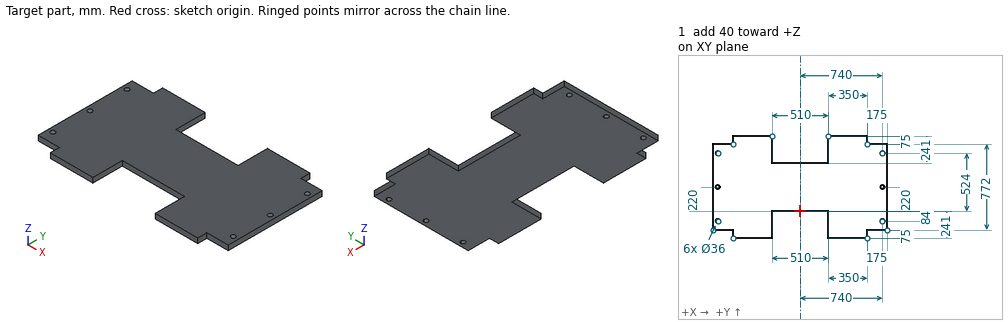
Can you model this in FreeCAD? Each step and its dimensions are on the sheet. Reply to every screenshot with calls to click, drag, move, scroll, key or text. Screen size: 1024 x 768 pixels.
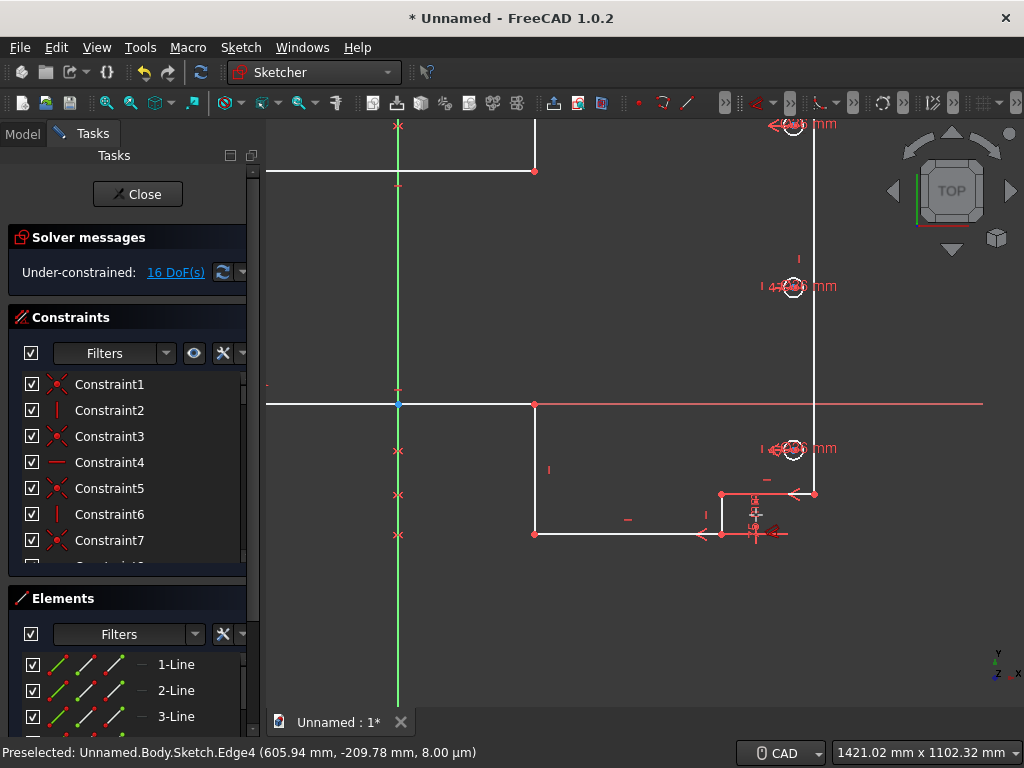
scroll(722, 516, down, 4)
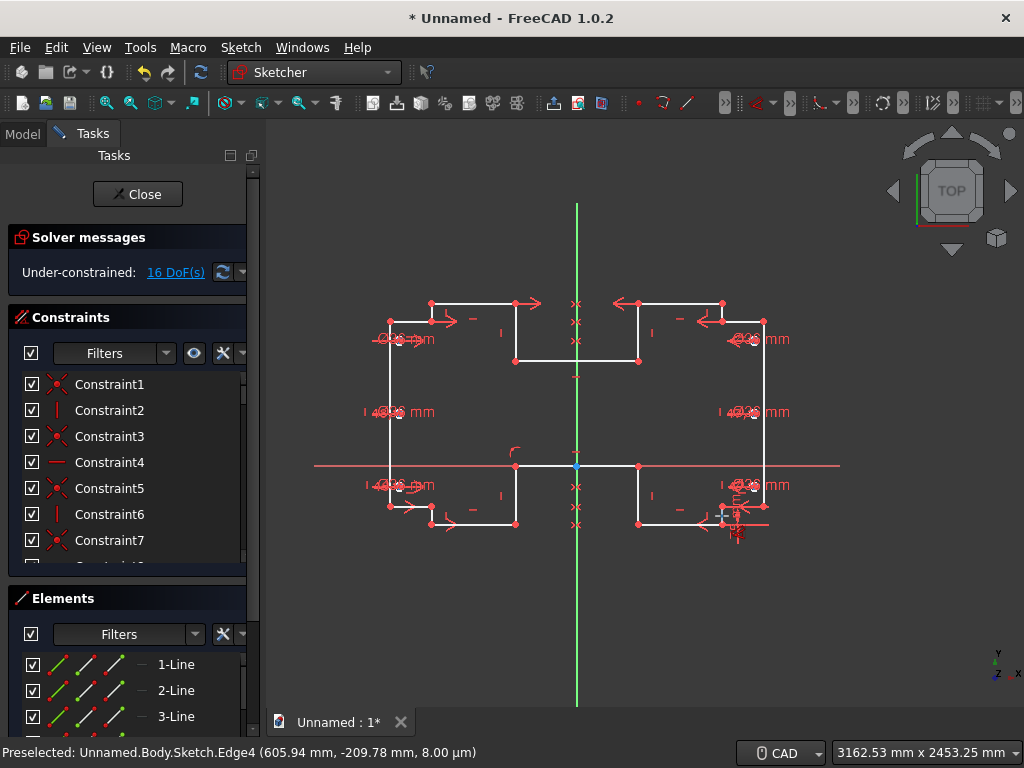
scroll(722, 316, up, 5)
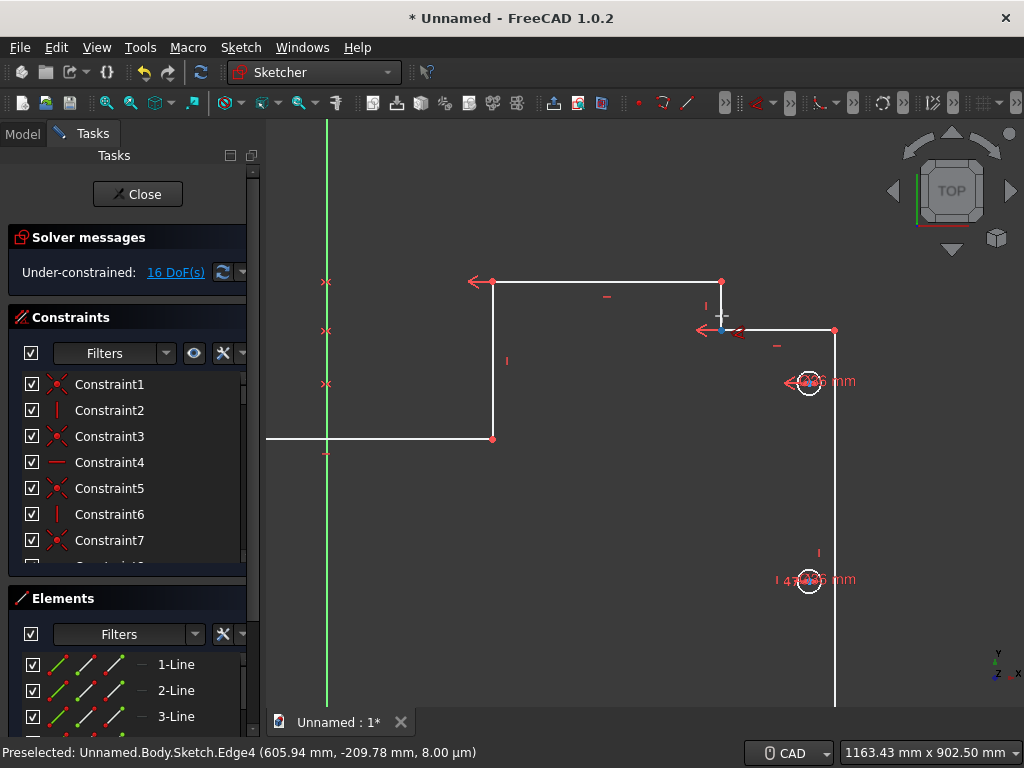
click(721, 316)
click(755, 306)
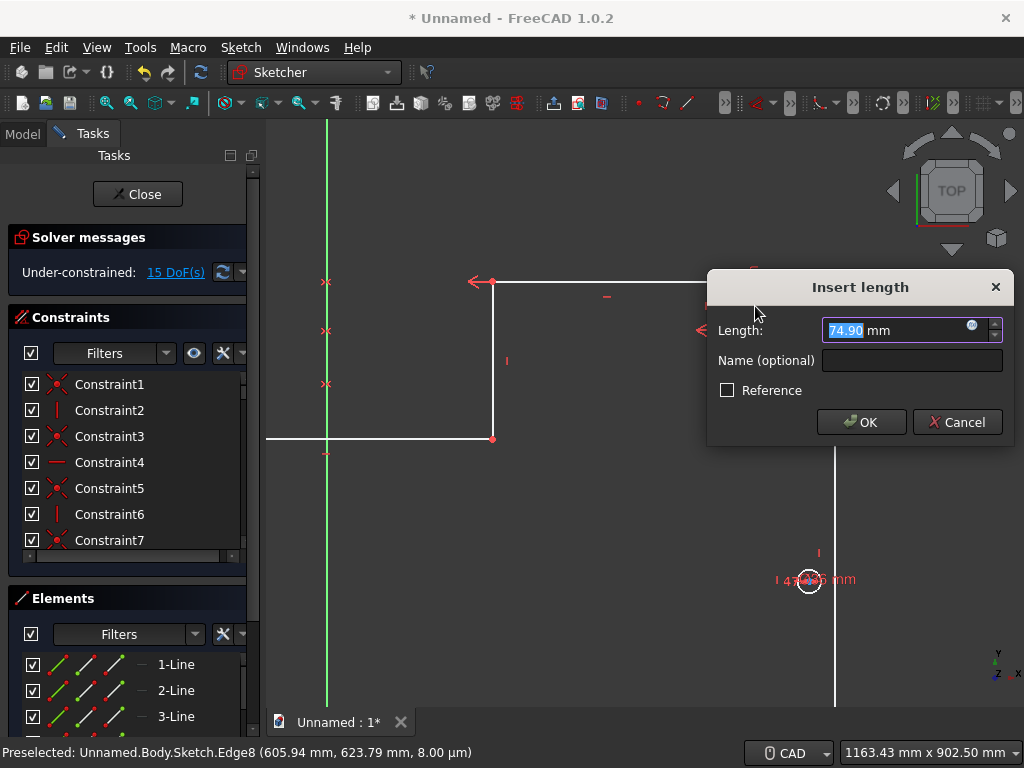
text(75)
key(Return)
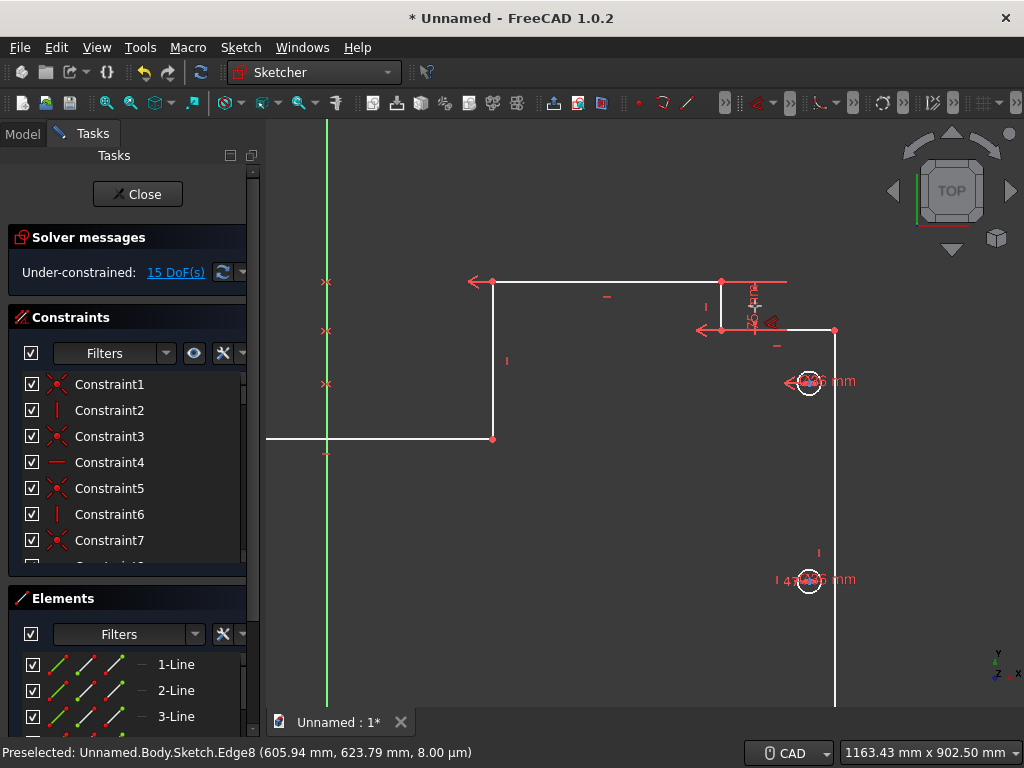
scroll(722, 316, down, 5)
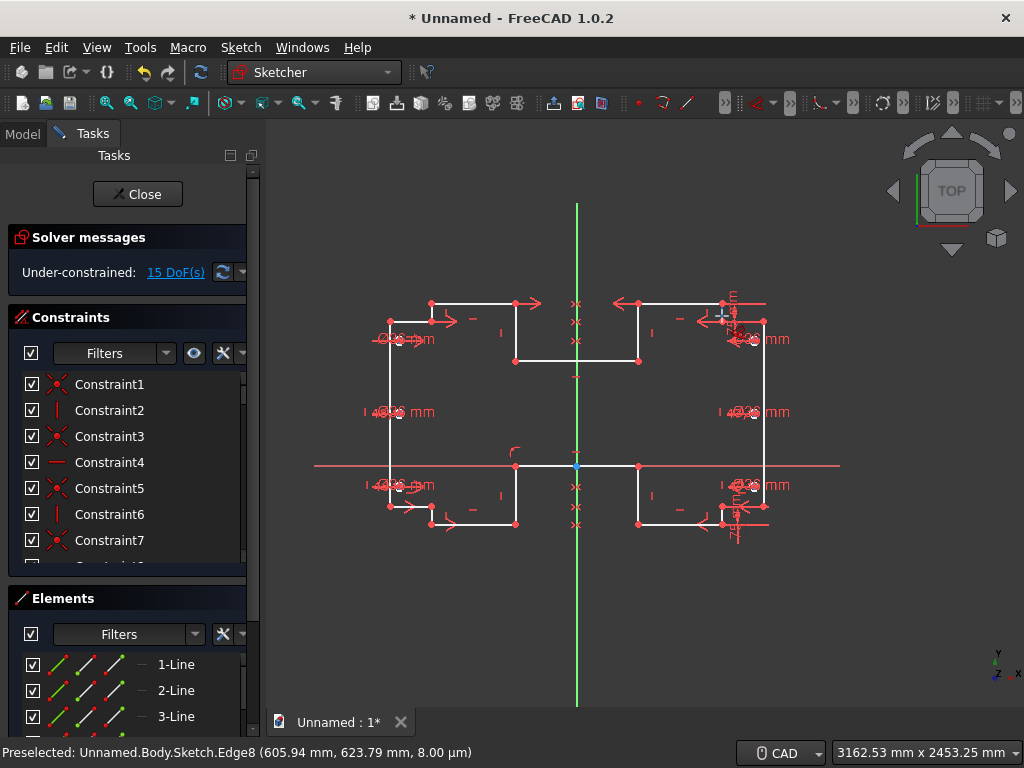
scroll(754, 487, up, 4)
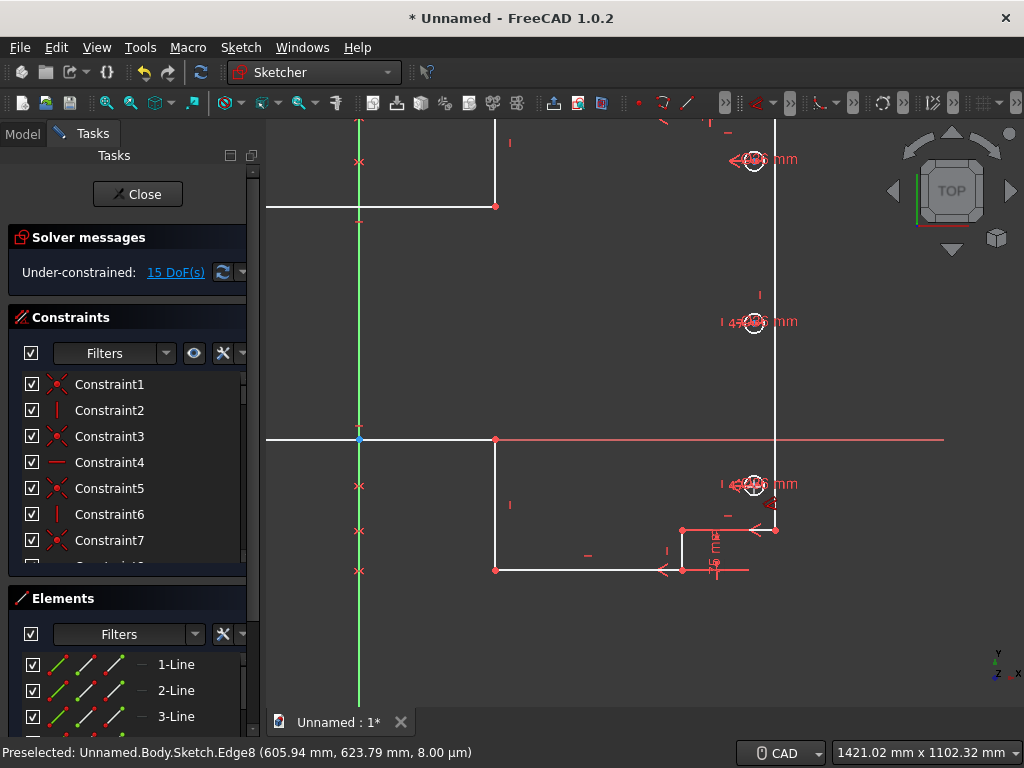
click(754, 486)
click(788, 463)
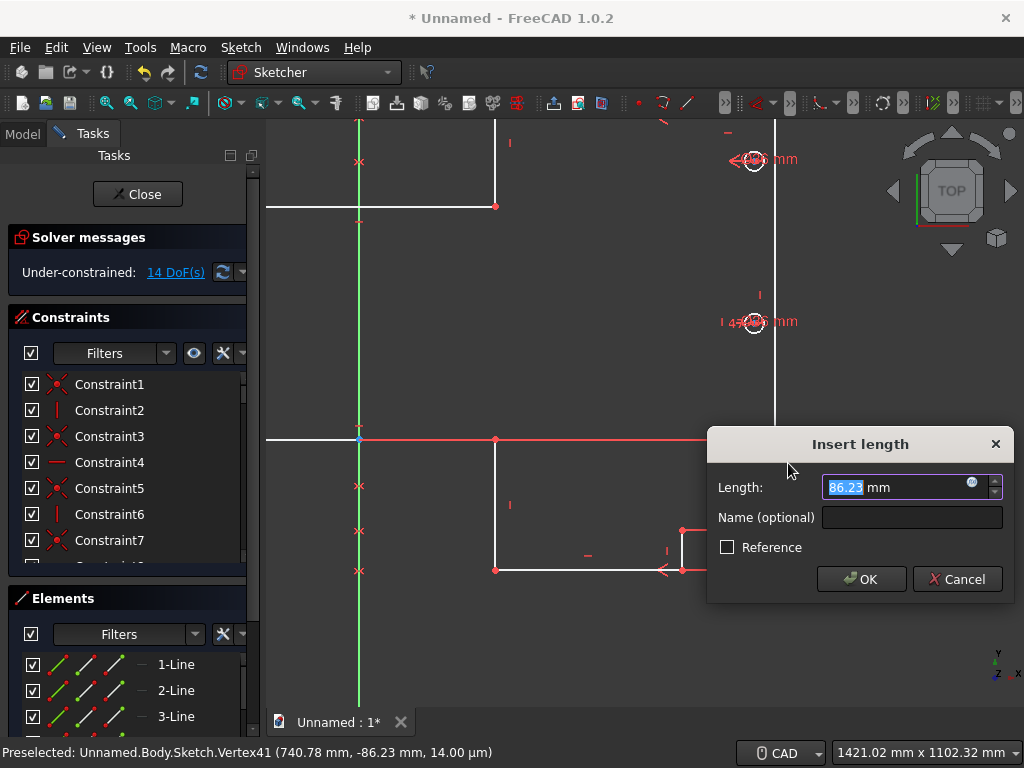
text(84)
key(Return)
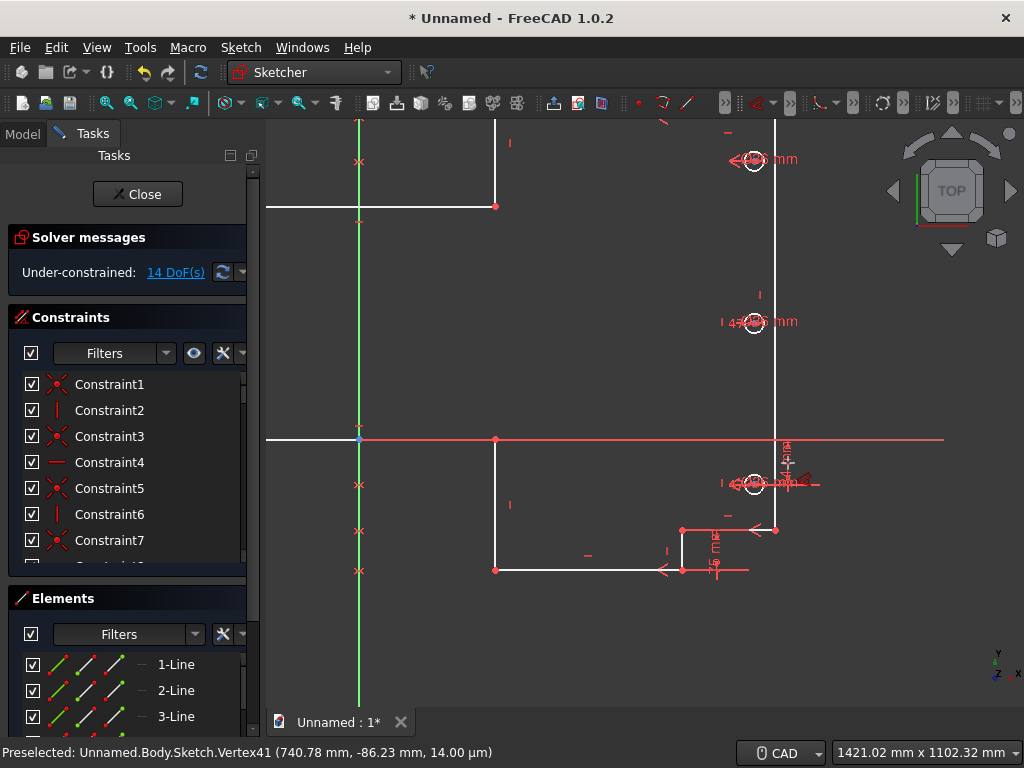
click(305, 440)
click(395, 474)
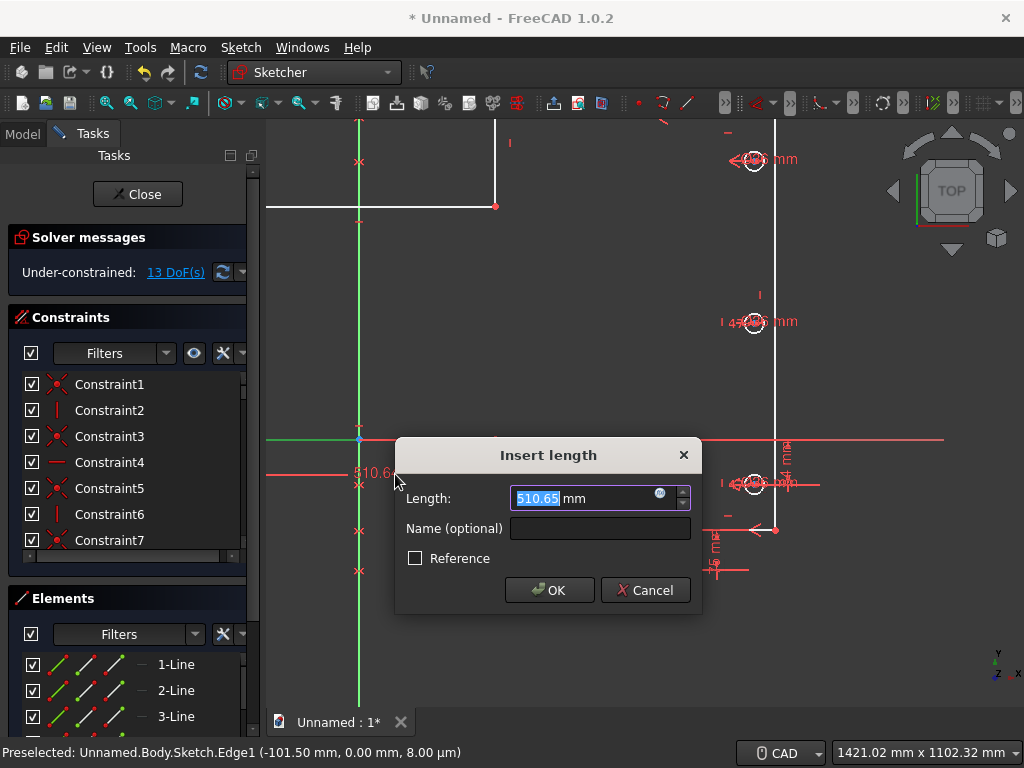
text(510)
key(Return)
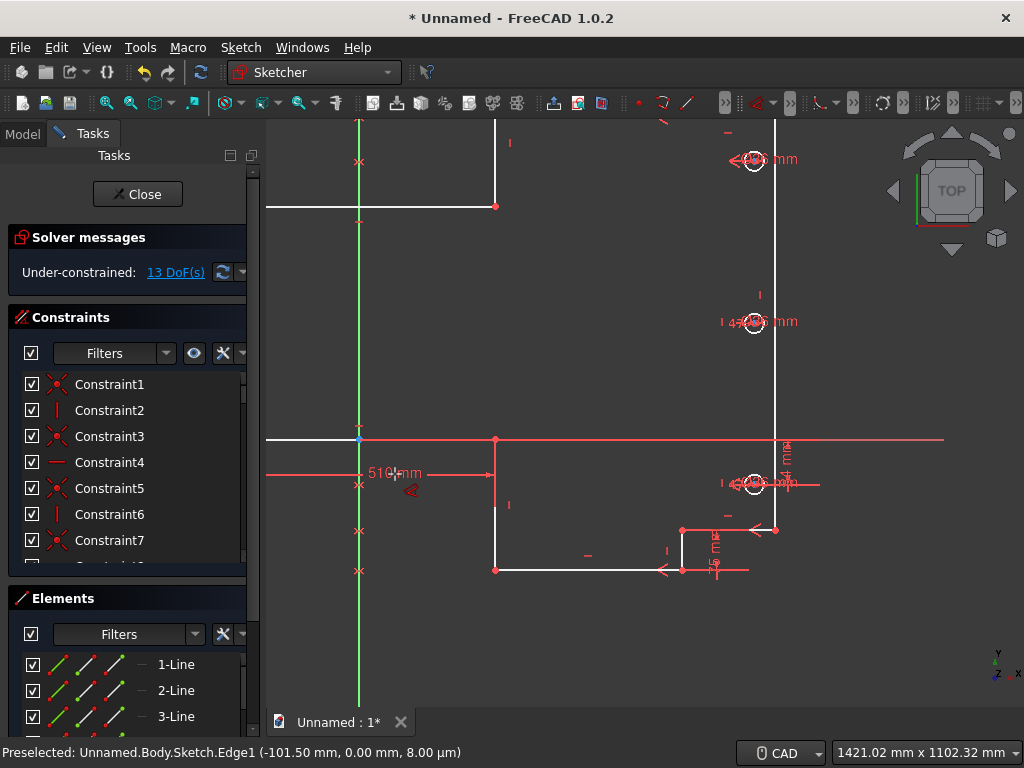
click(495, 479)
click(529, 505)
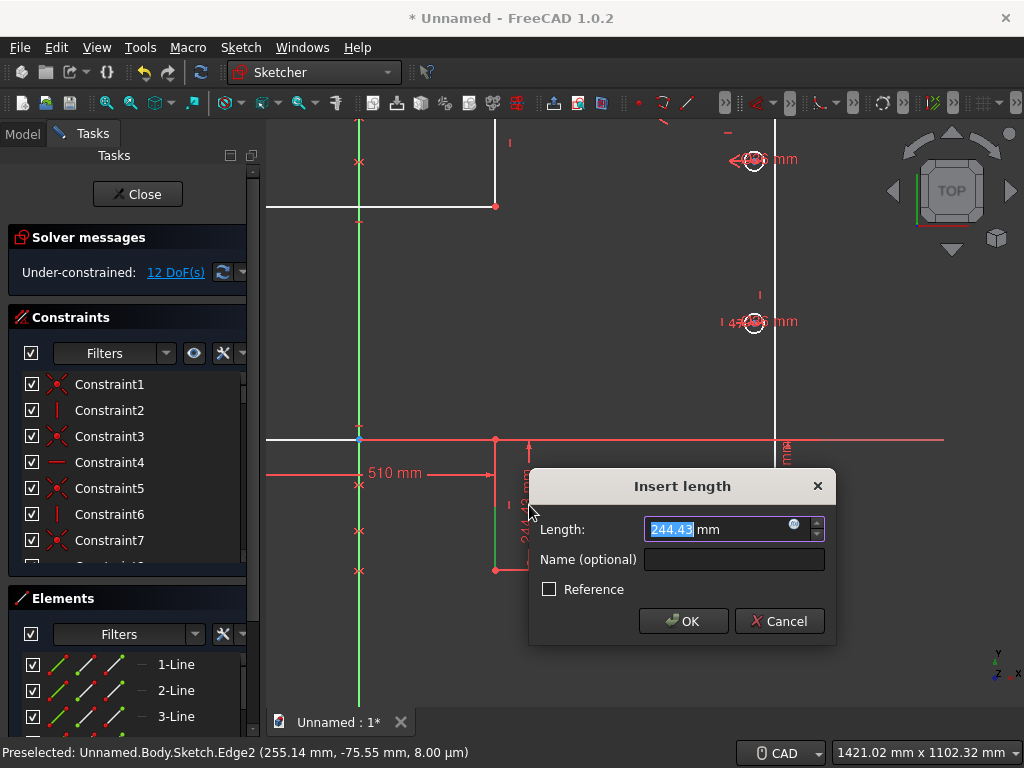
text(241)
key(Return)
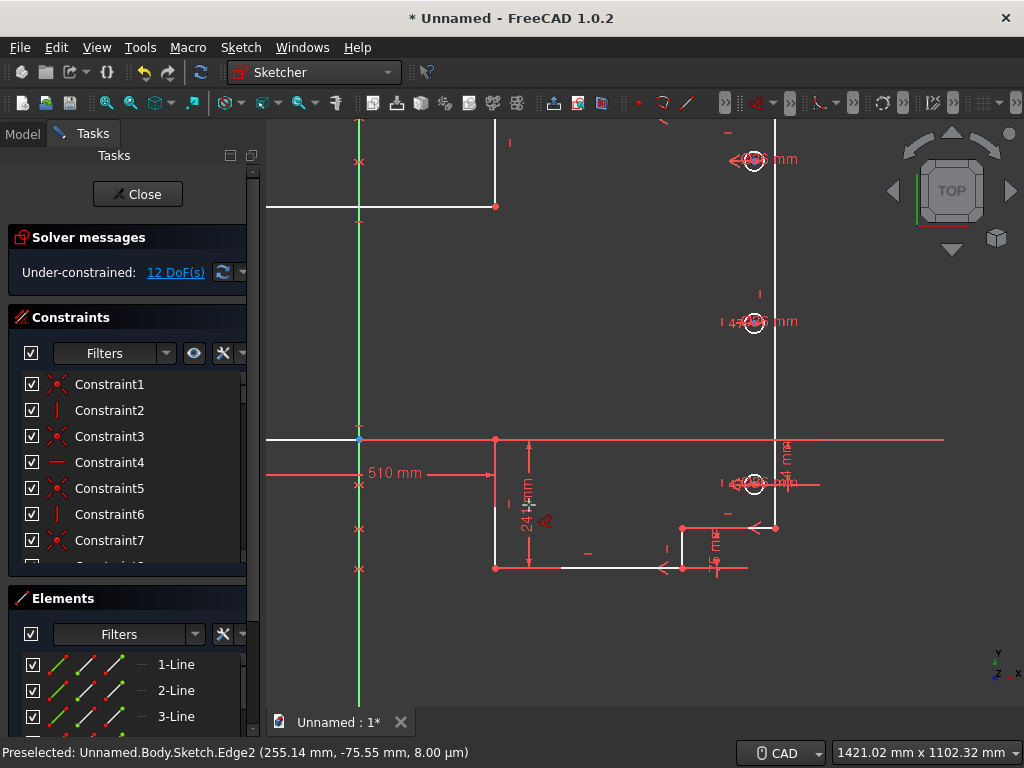
click(551, 568)
click(589, 602)